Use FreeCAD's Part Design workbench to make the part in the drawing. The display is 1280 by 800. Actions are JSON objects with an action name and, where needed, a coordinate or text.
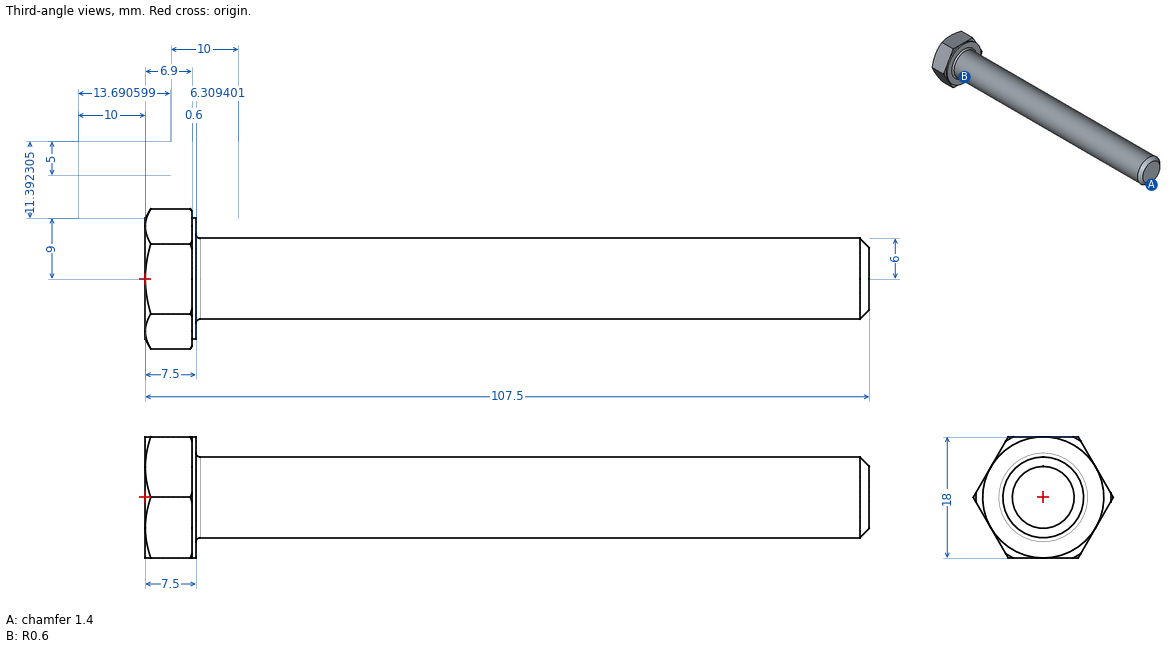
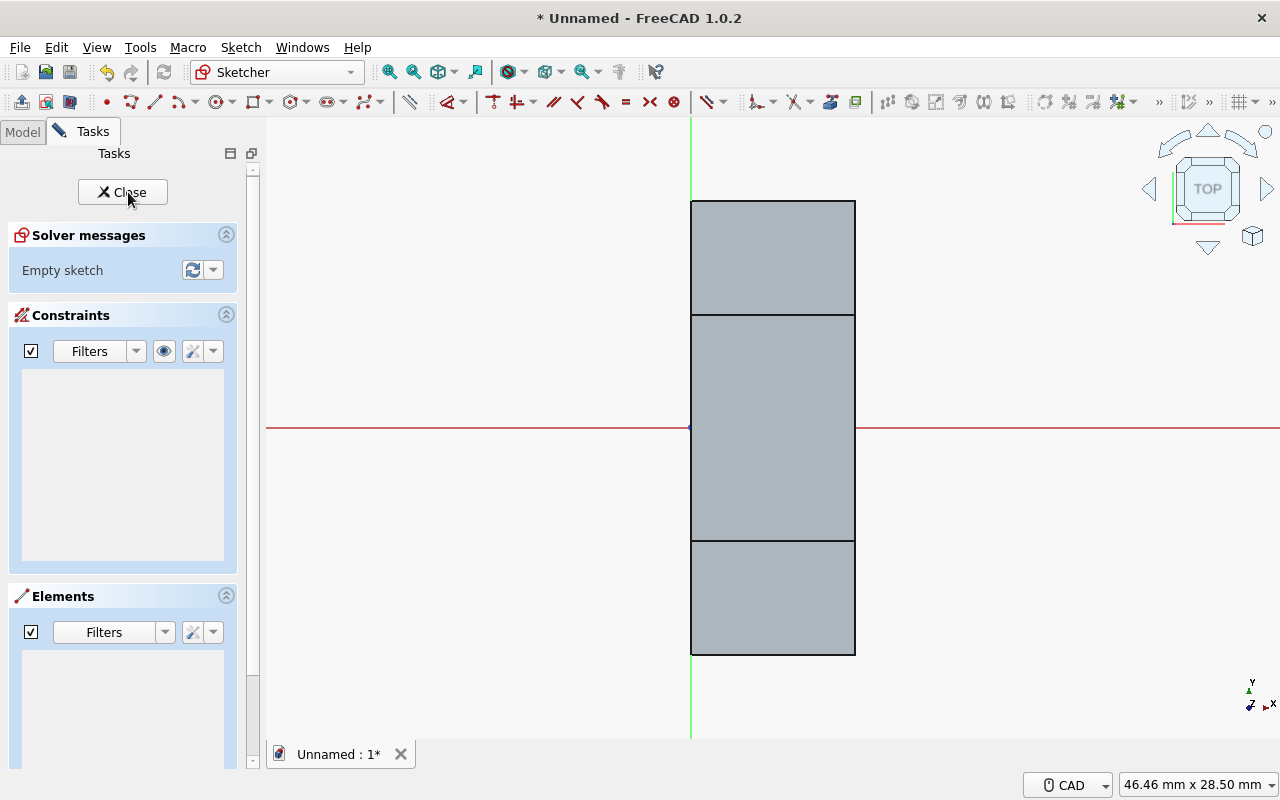
{"action": "key", "text": "q s"}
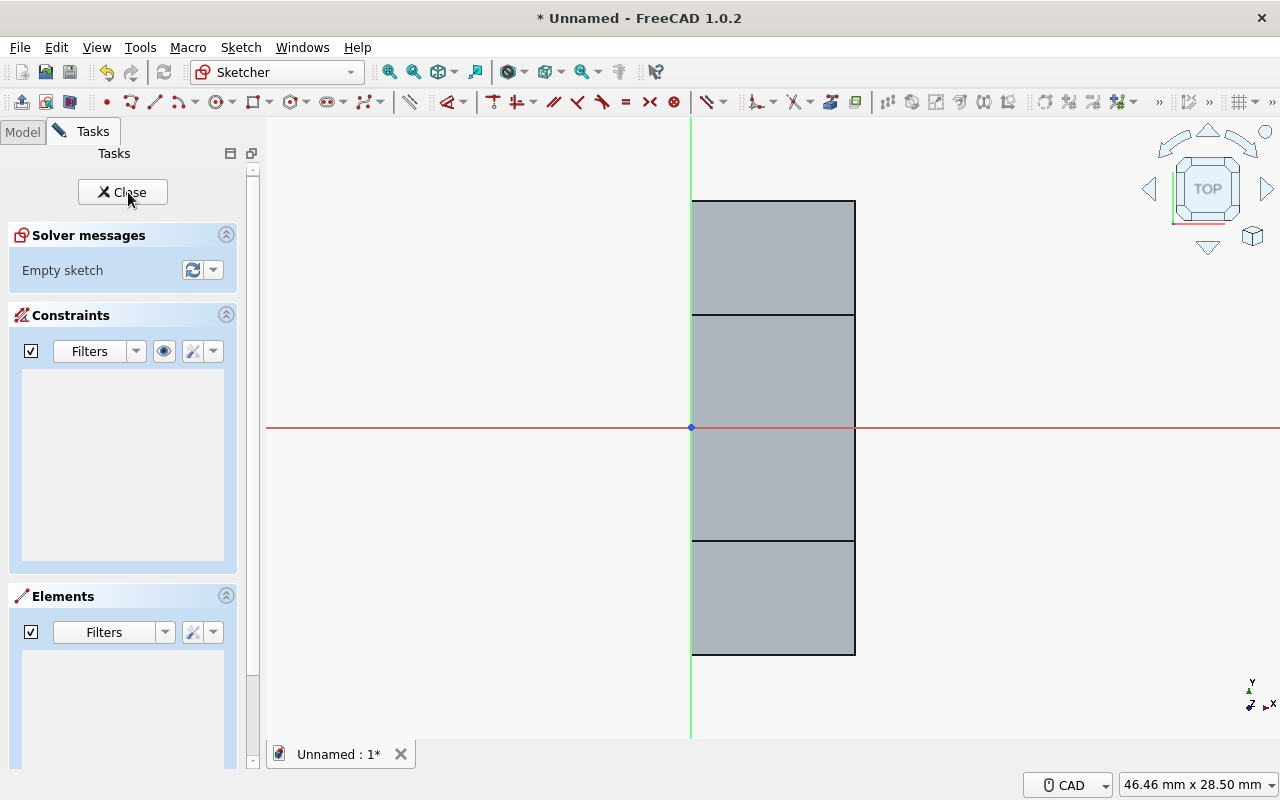
{"action": "scroll", "coordinate": [325, 449], "scroll_direction": "down", "scroll_amount": 7}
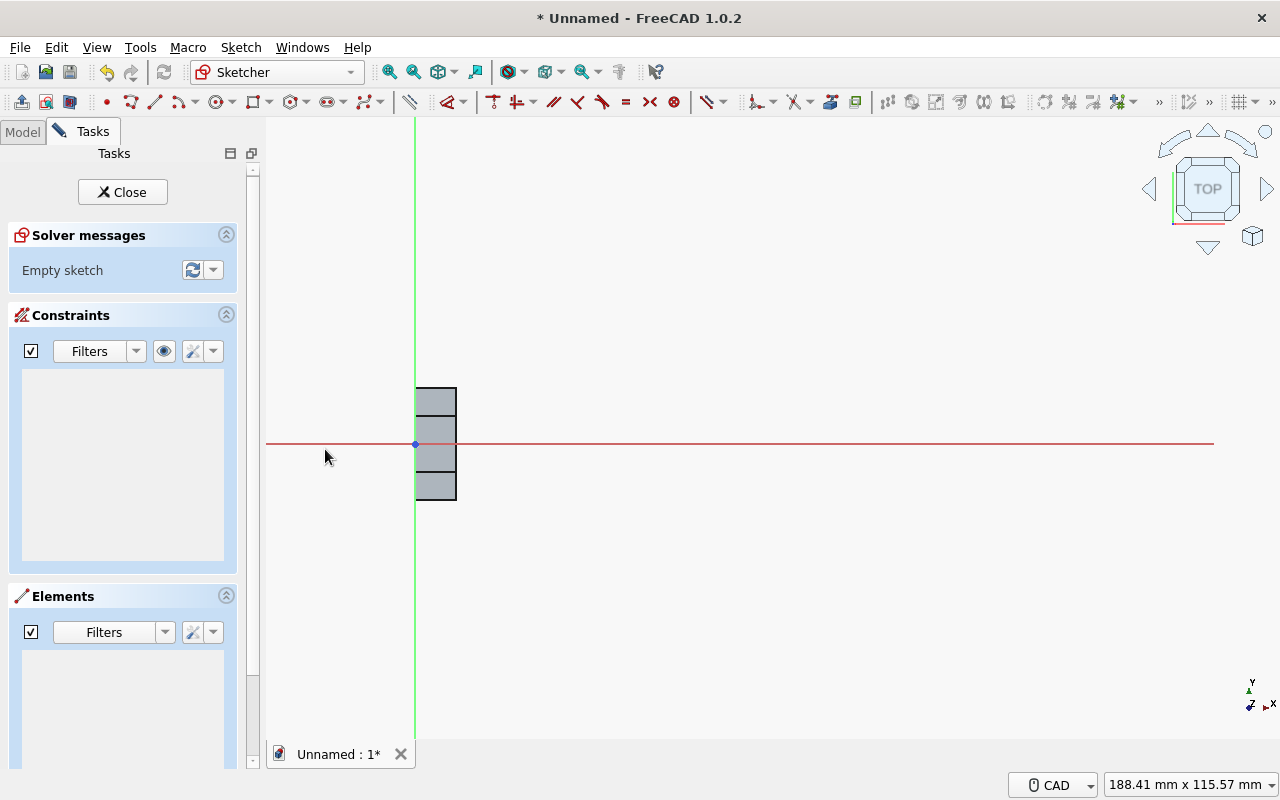
{"action": "key", "text": "g r"}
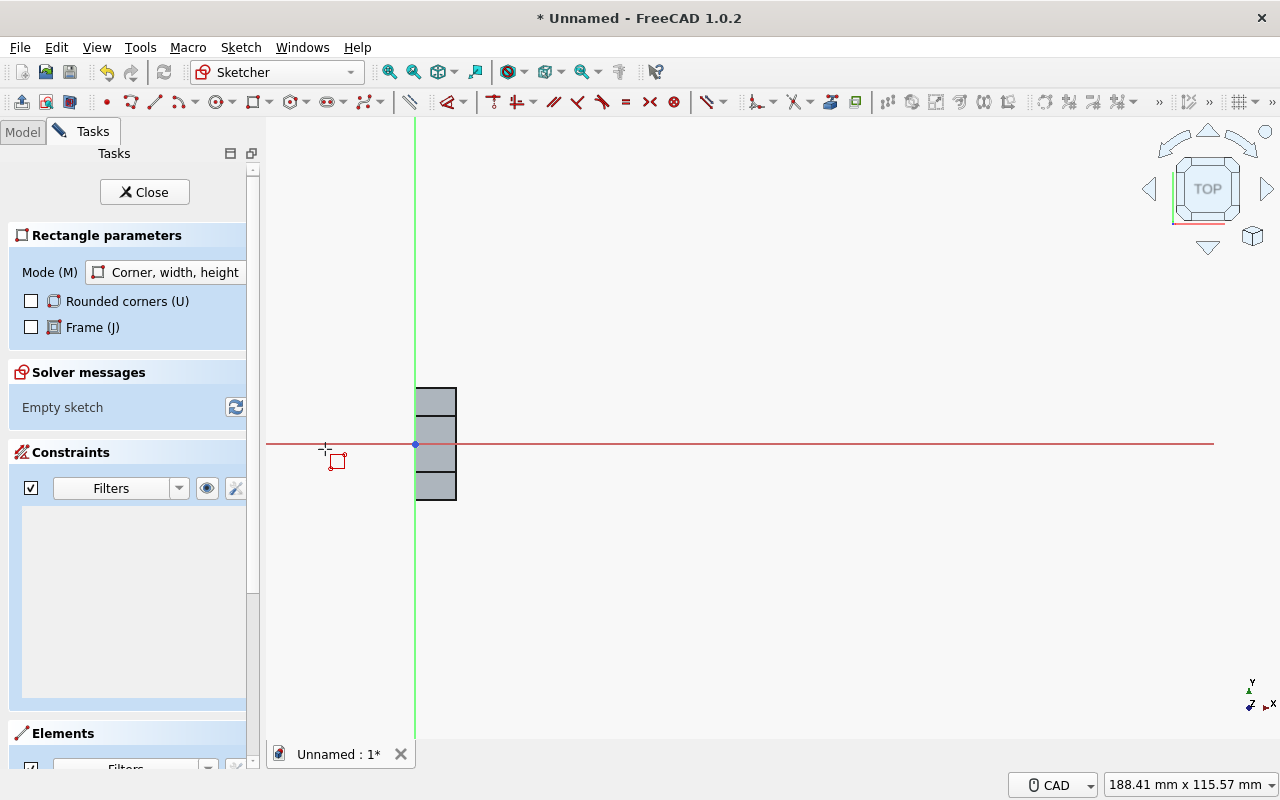
{"action": "left_click", "coordinate": [415, 444]}
{"action": "mouse_move", "coordinate": [994, 412]}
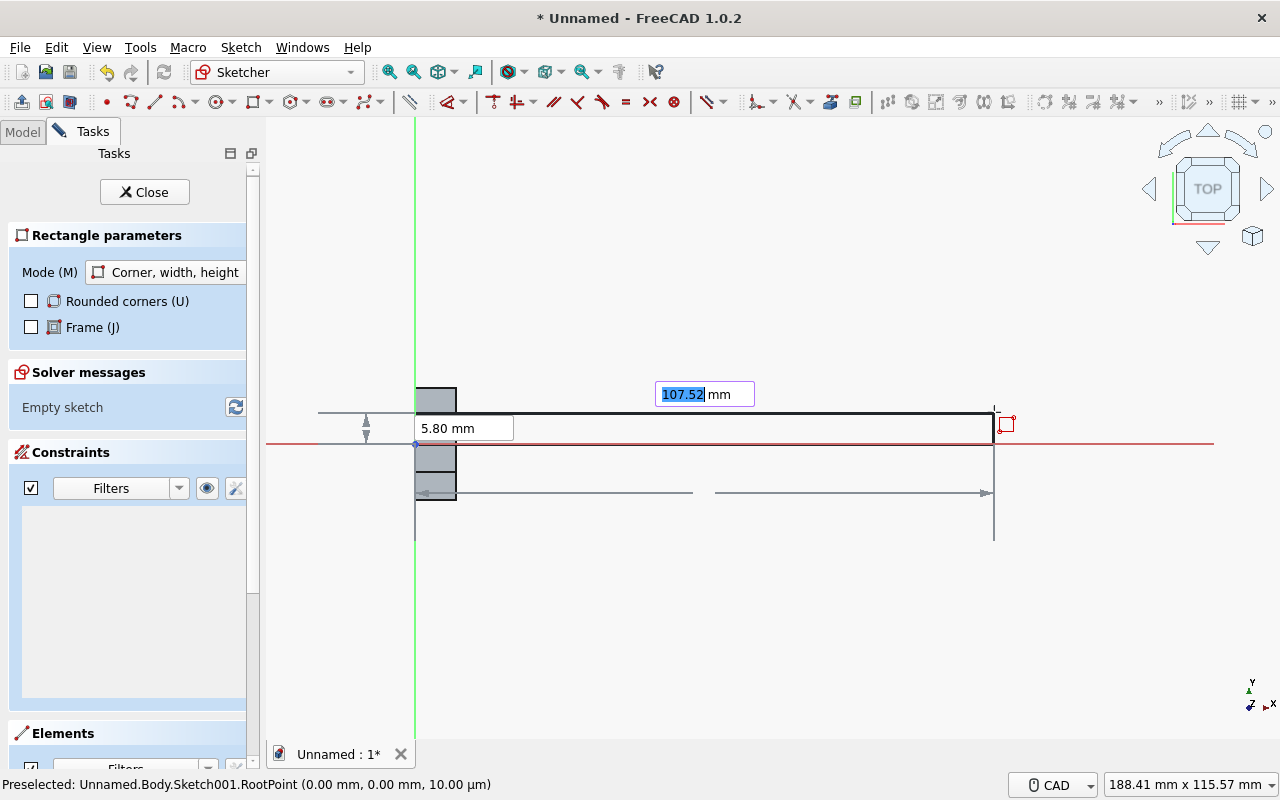
{"action": "type", "text": "107.5"}
{"action": "key", "text": "Tab"}
{"action": "type", "text": "6"}
{"action": "key", "text": "Return"}
{"action": "key", "text": "Escape"}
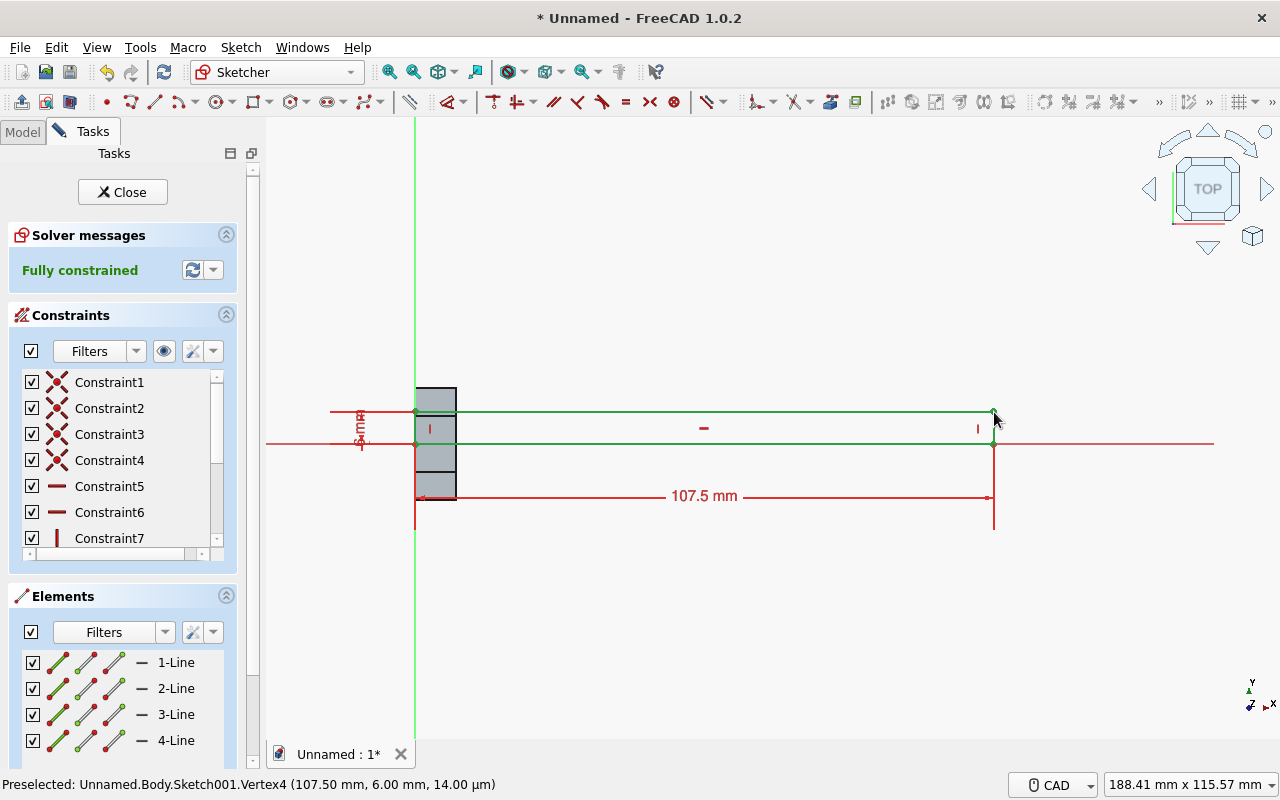
{"action": "left_click", "coordinate": [123, 192]}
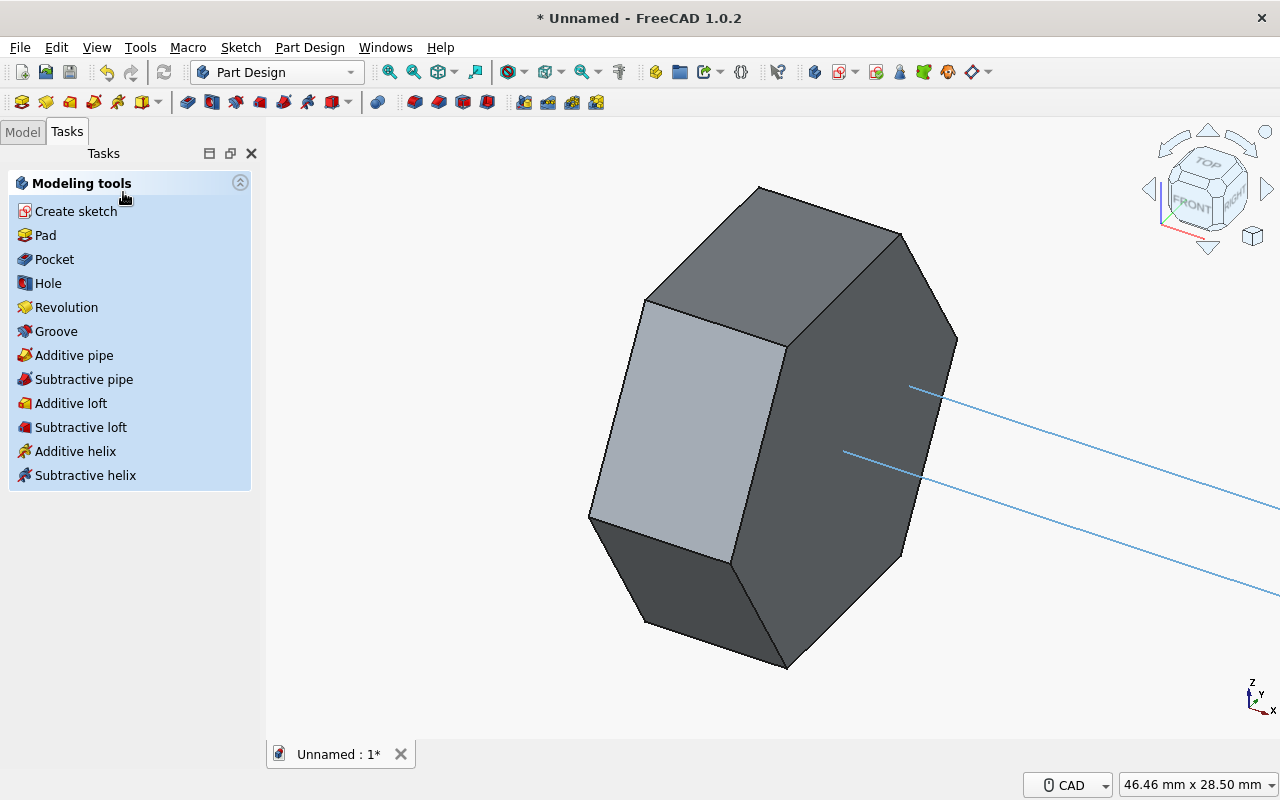
{"action": "left_click", "coordinate": [46, 102]}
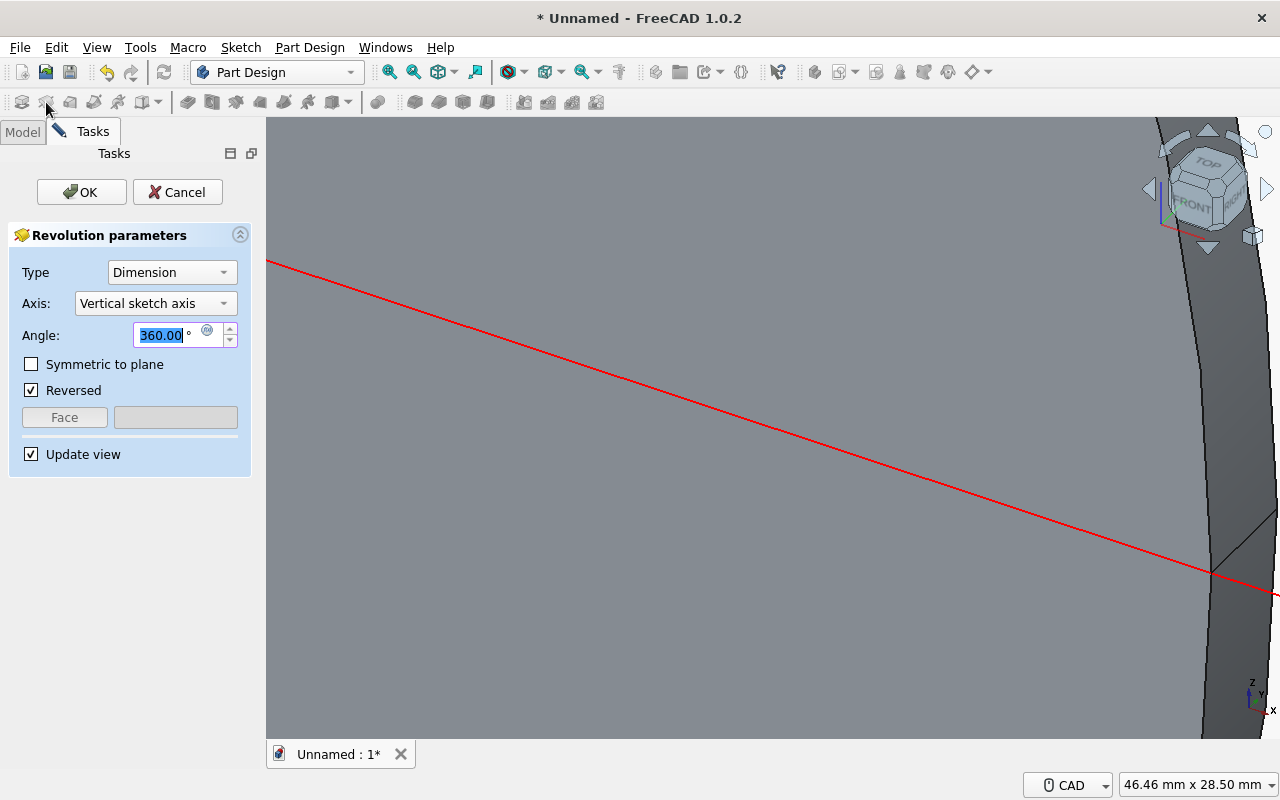
{"action": "left_click", "coordinate": [156, 304]}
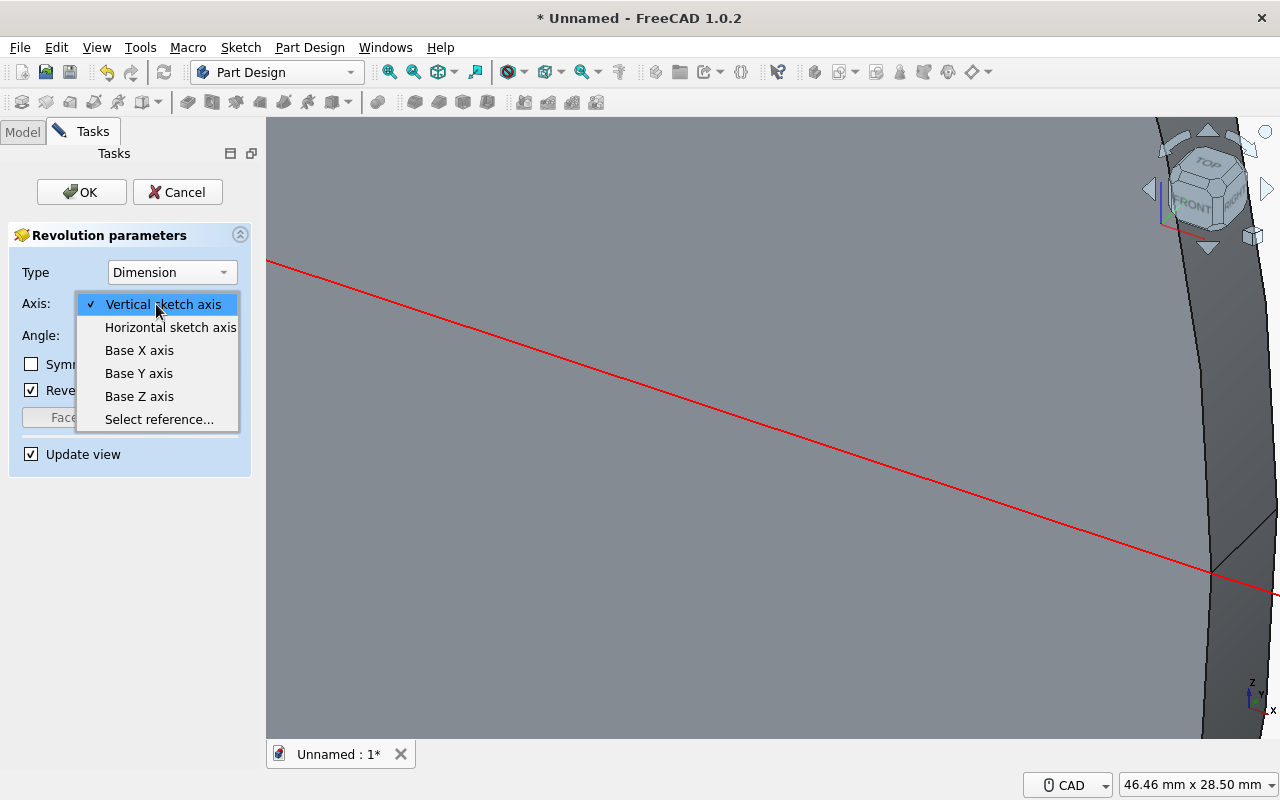
{"action": "left_click", "coordinate": [156, 328]}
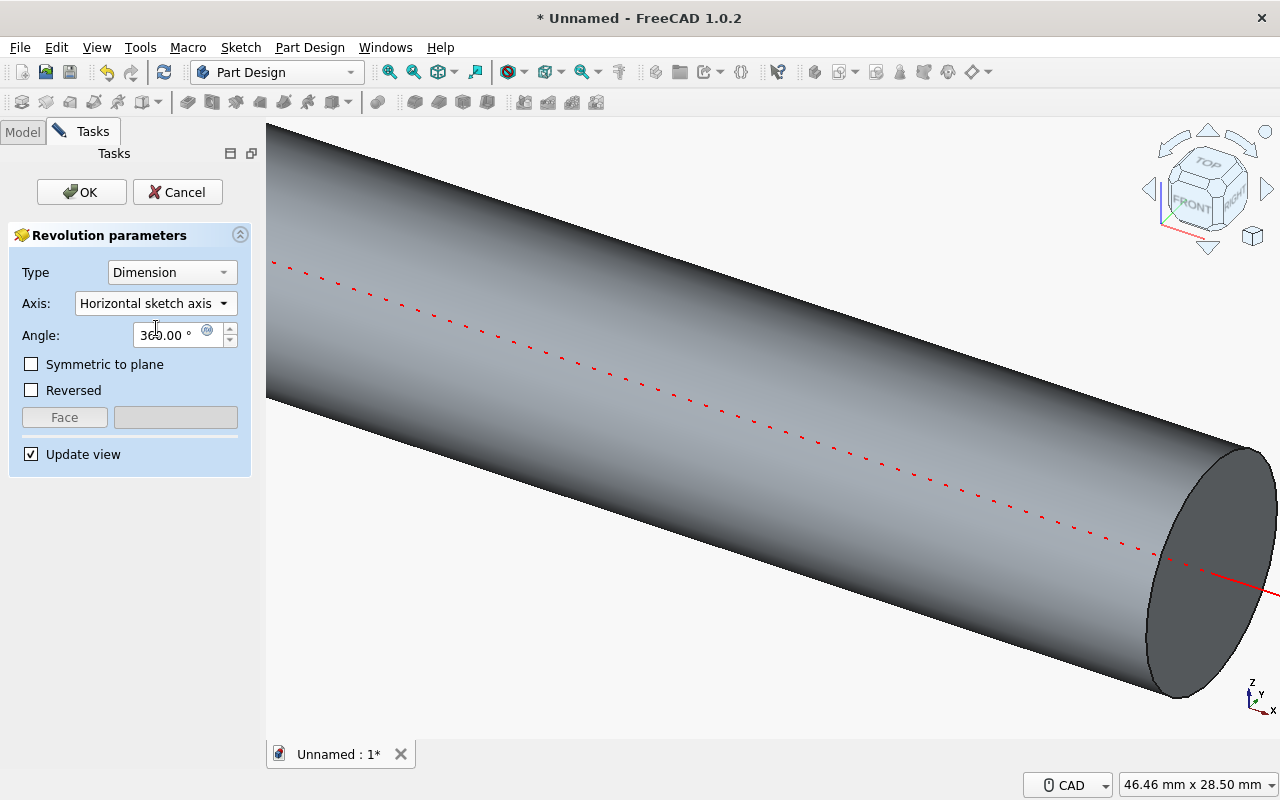
{"action": "left_click", "coordinate": [82, 192]}